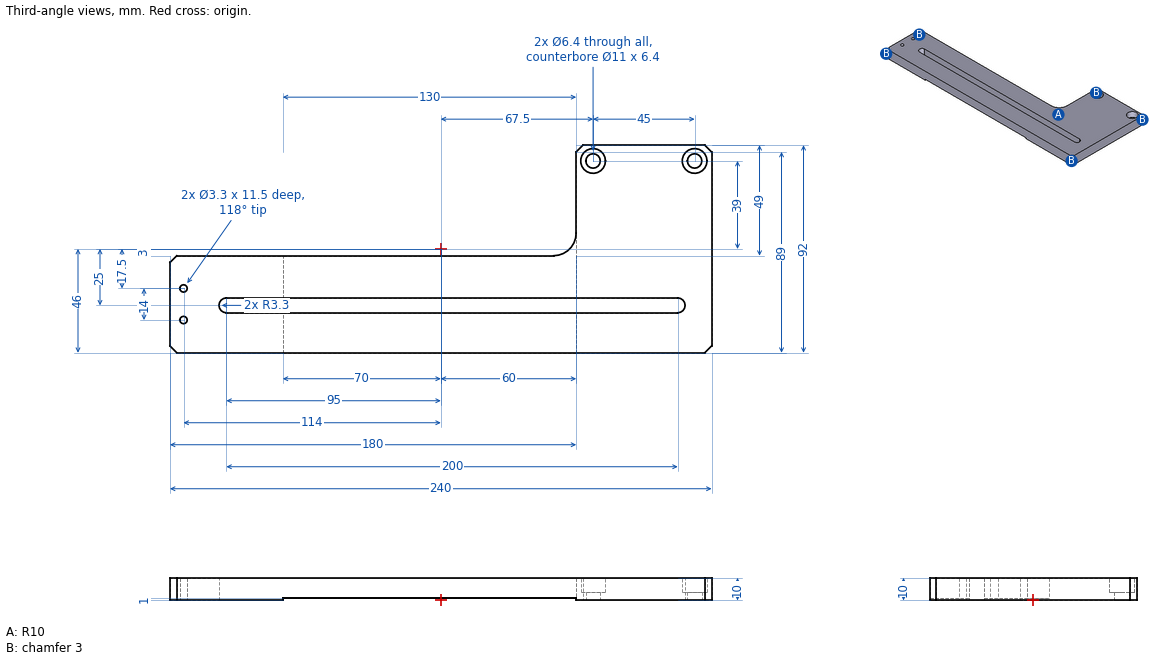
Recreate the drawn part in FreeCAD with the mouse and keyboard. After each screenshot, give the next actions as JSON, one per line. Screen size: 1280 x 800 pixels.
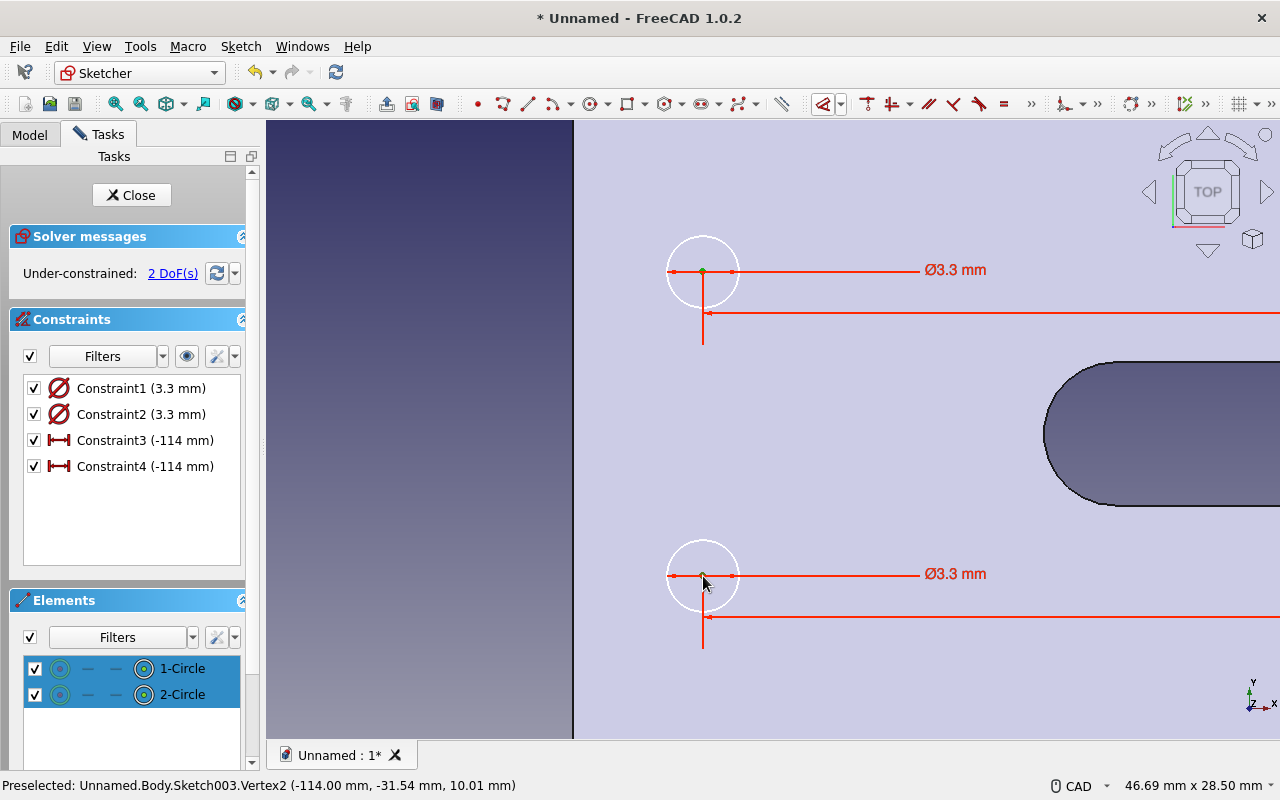
{"action": "key", "text": "i"}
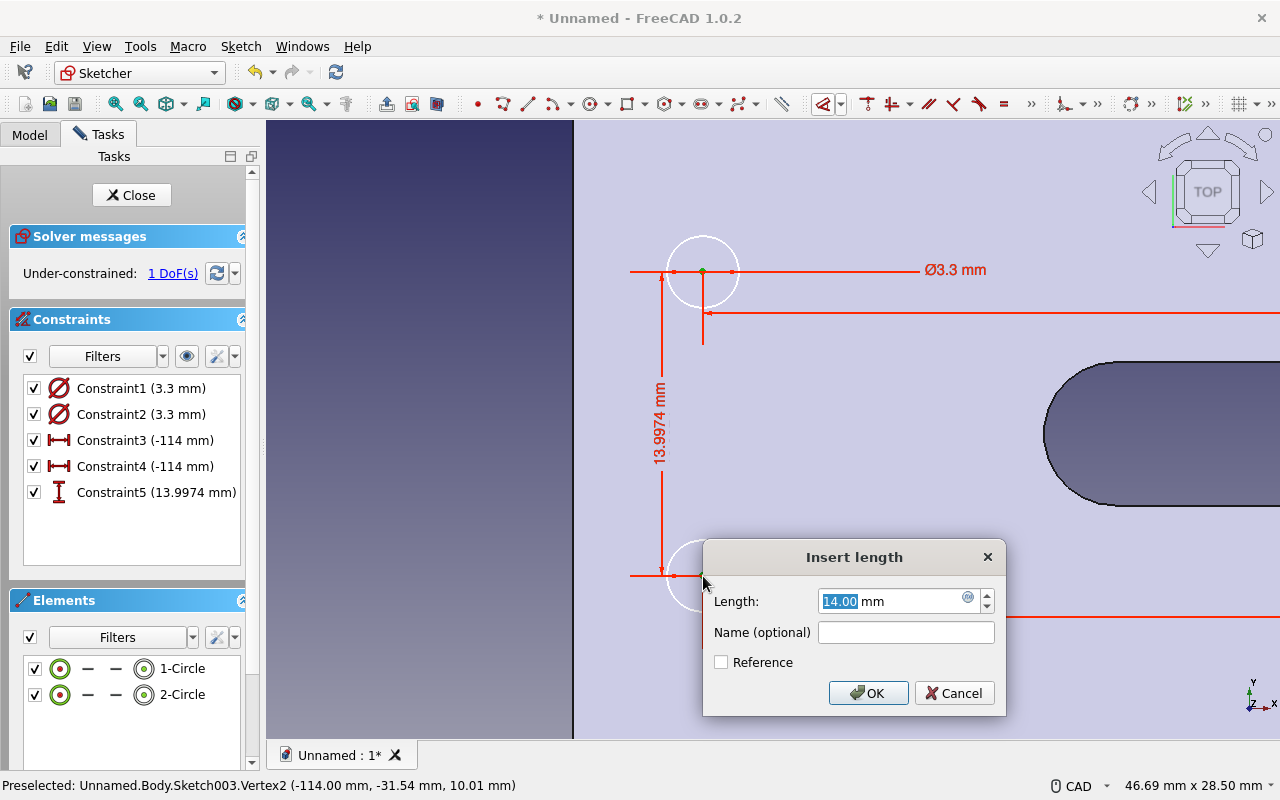
{"action": "type", "text": "14"}
{"action": "key", "text": "Return"}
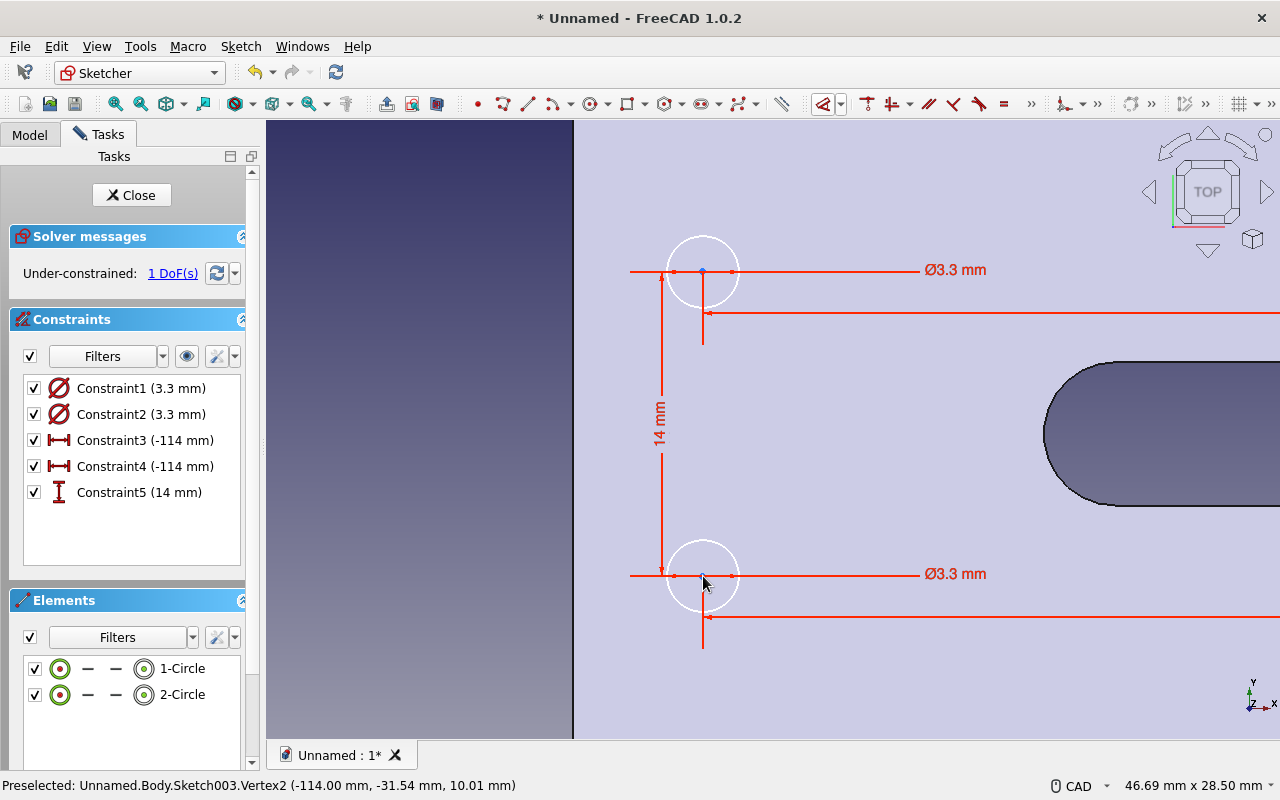
{"action": "left_click", "coordinate": [703, 272]}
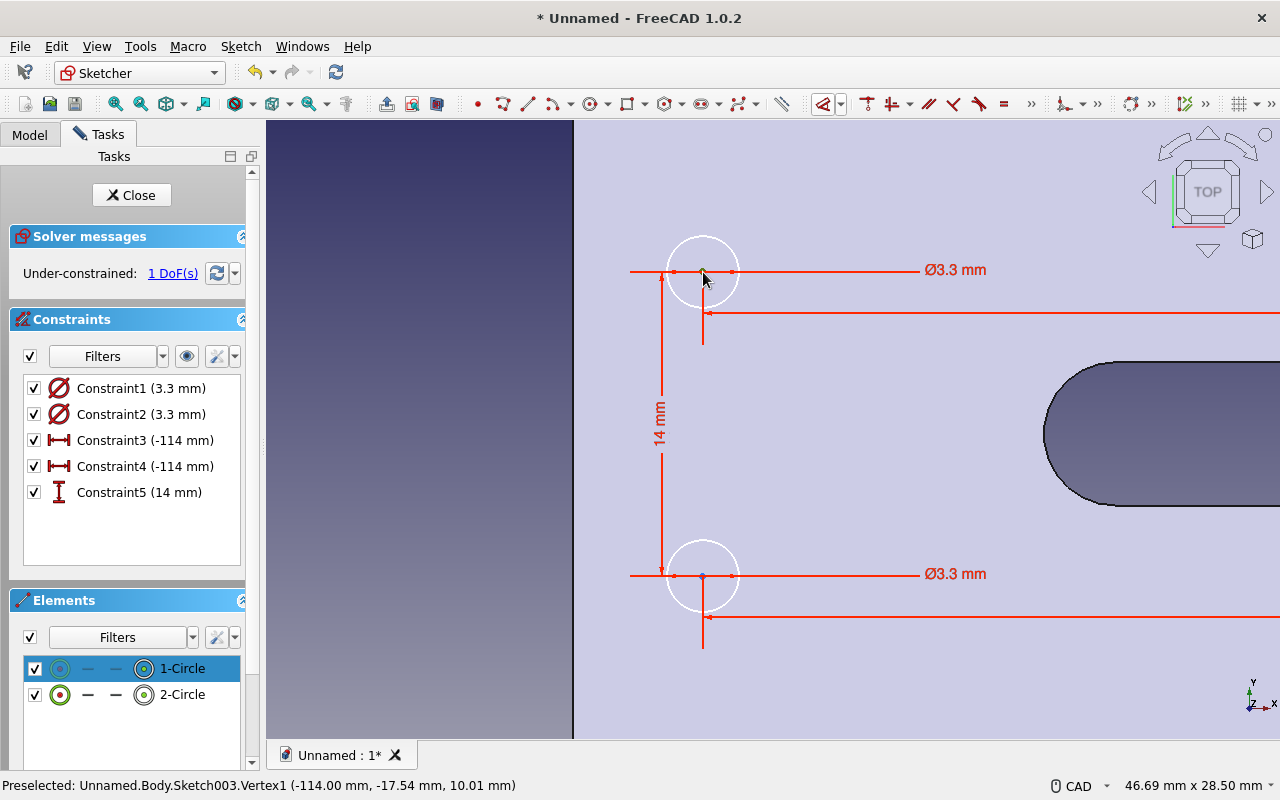
{"action": "key", "text": "i"}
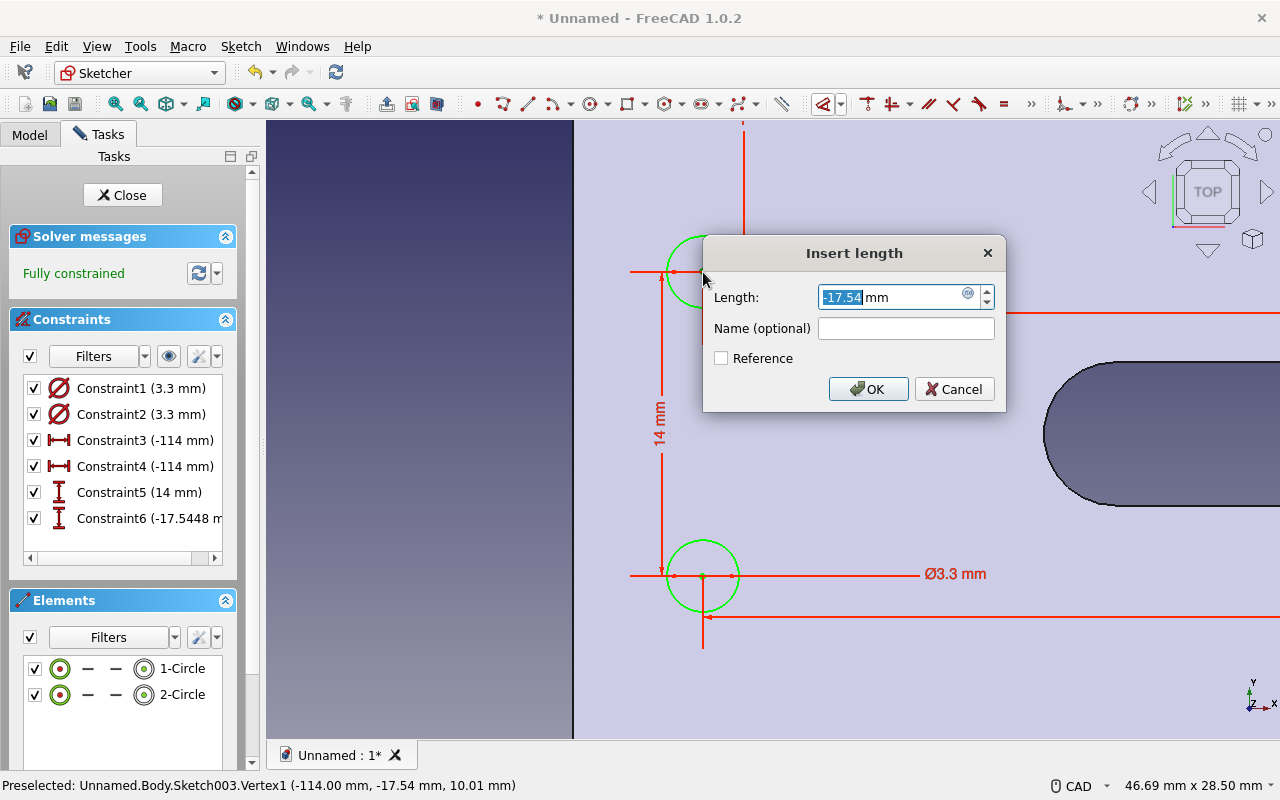
{"action": "type", "text": "-17.5"}
{"action": "key", "text": "Return"}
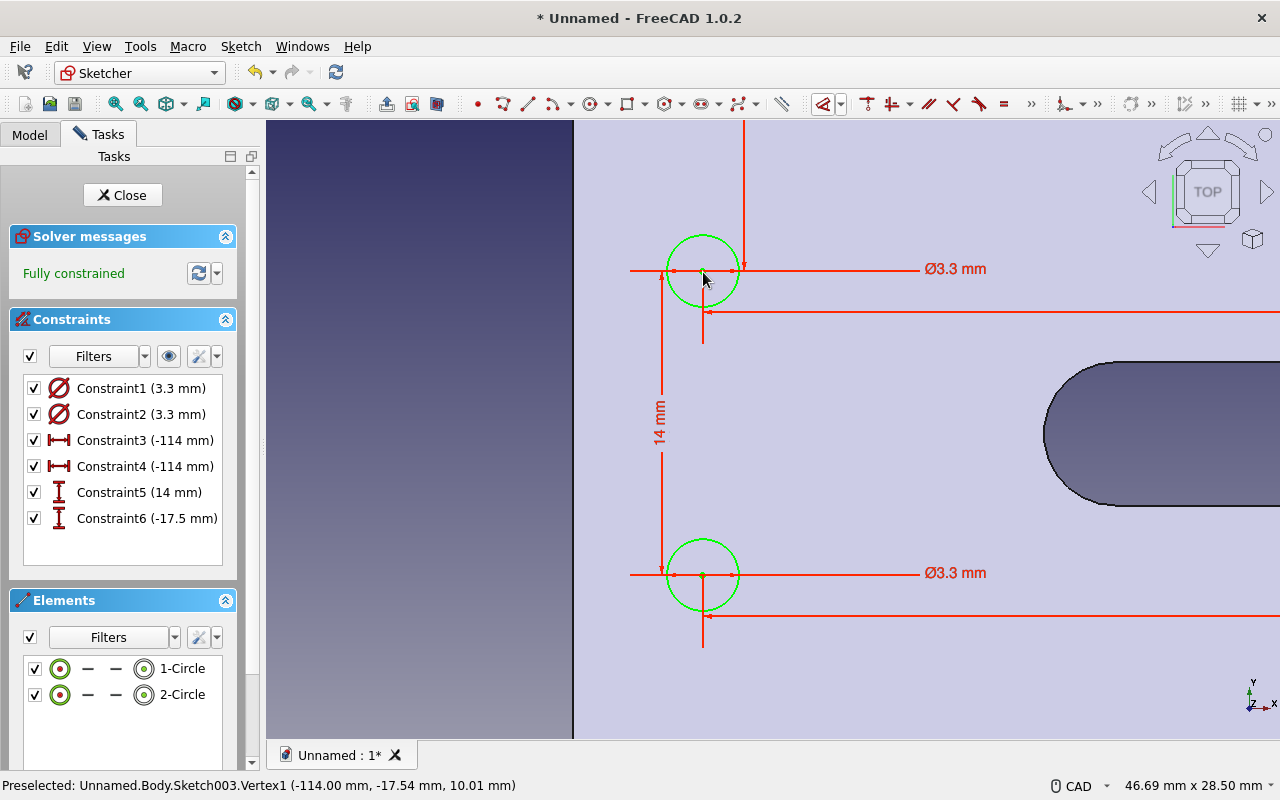
{"action": "left_click", "coordinate": [123, 195]}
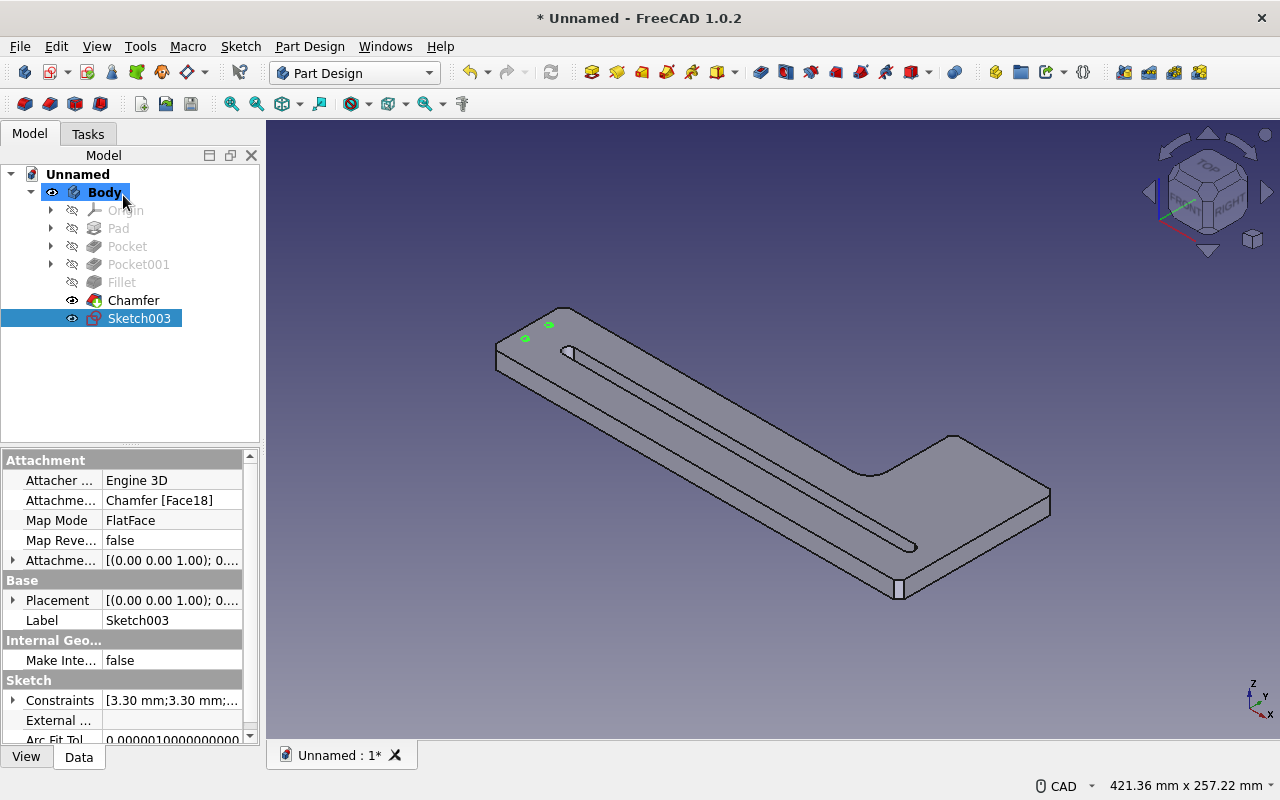
{"action": "left_click", "coordinate": [786, 72]}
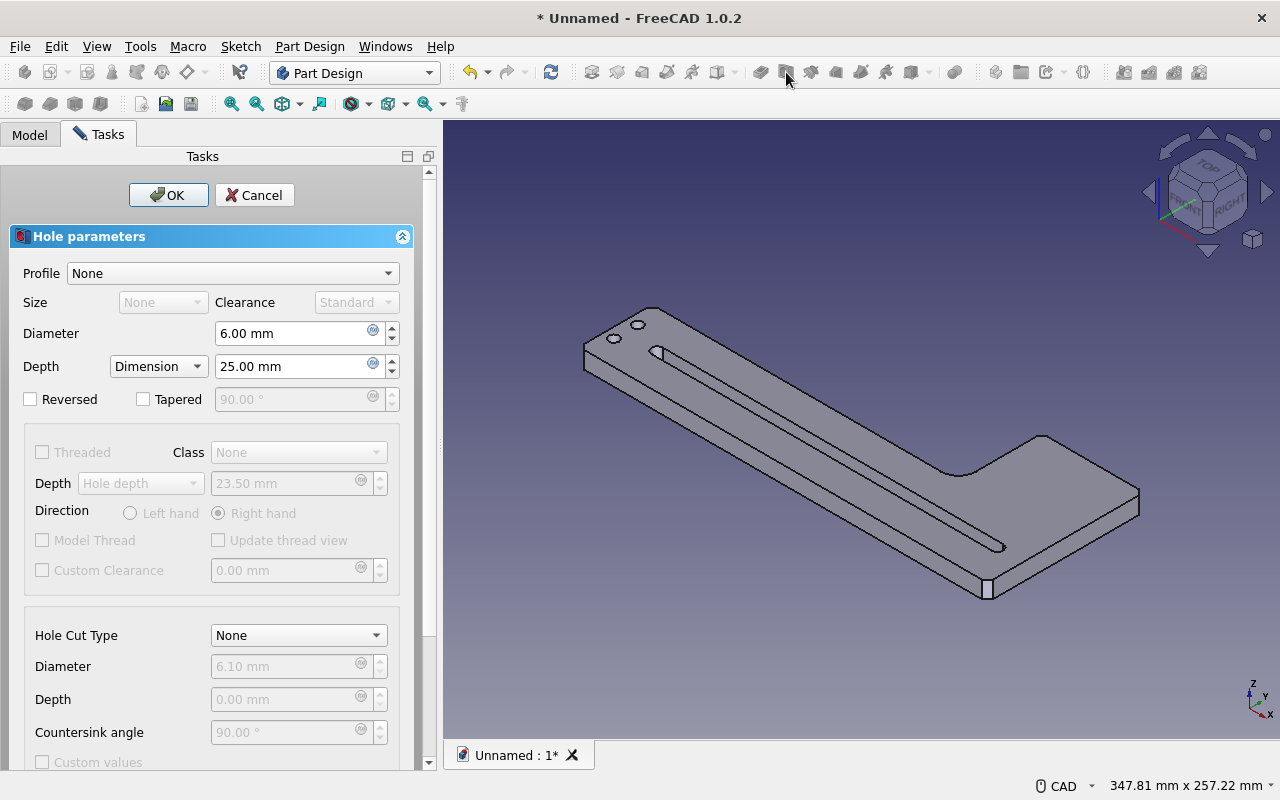
{"action": "triple_click", "coordinate": [300, 334]}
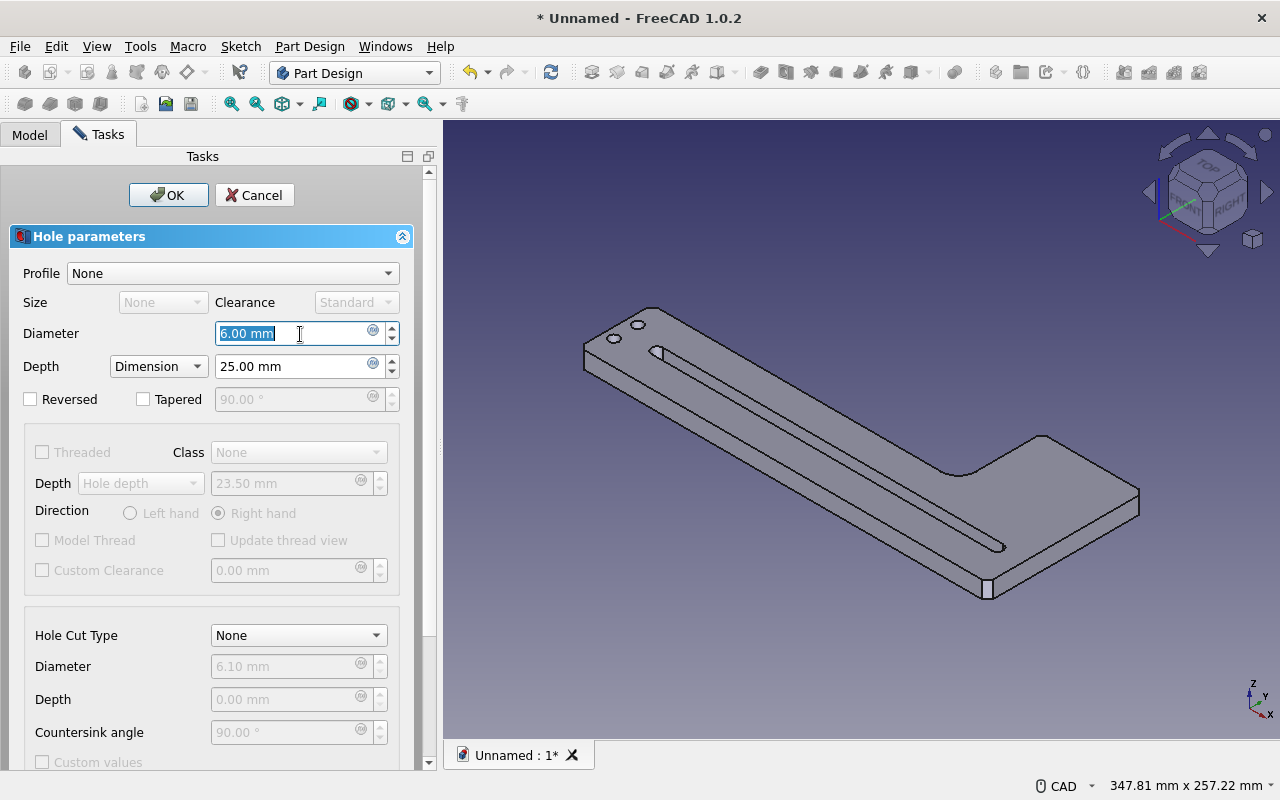
{"action": "type", "text": "3.3"}
{"action": "key", "text": "Tab"}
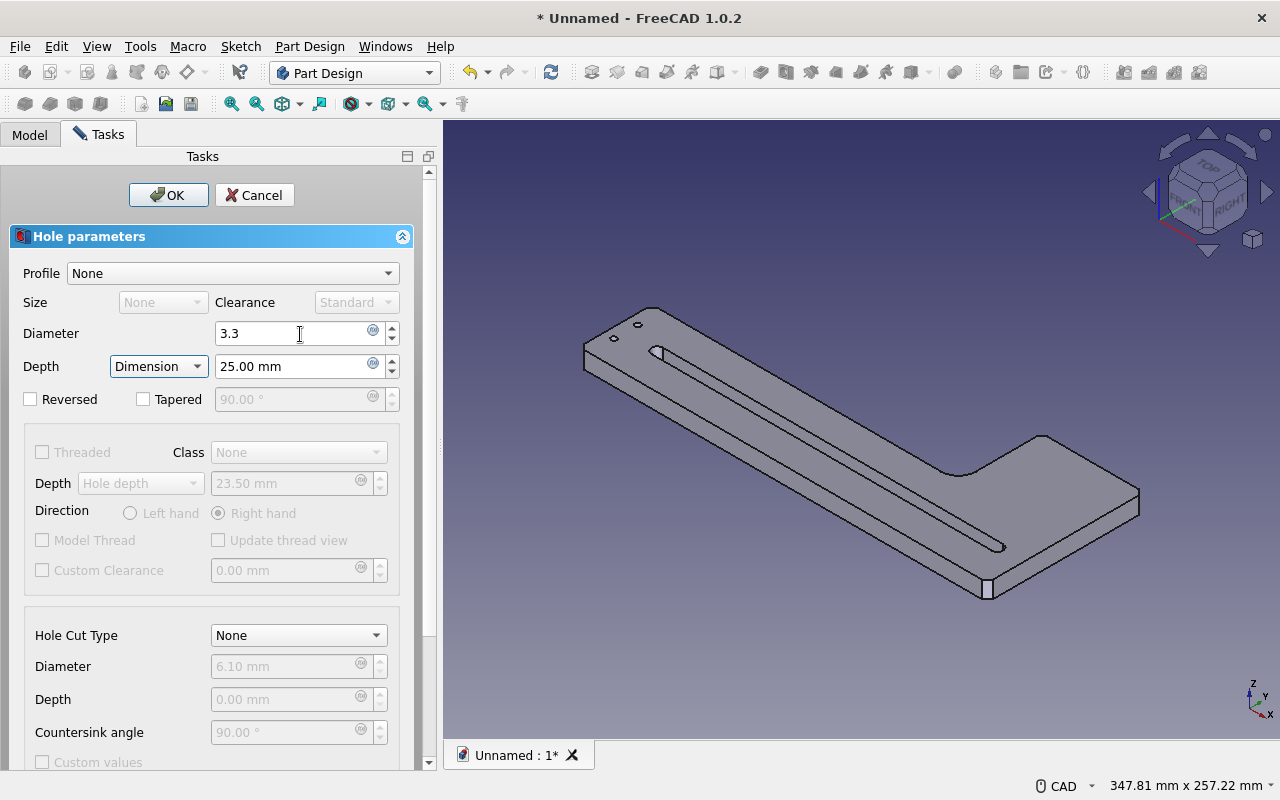
{"action": "triple_click", "coordinate": [300, 366]}